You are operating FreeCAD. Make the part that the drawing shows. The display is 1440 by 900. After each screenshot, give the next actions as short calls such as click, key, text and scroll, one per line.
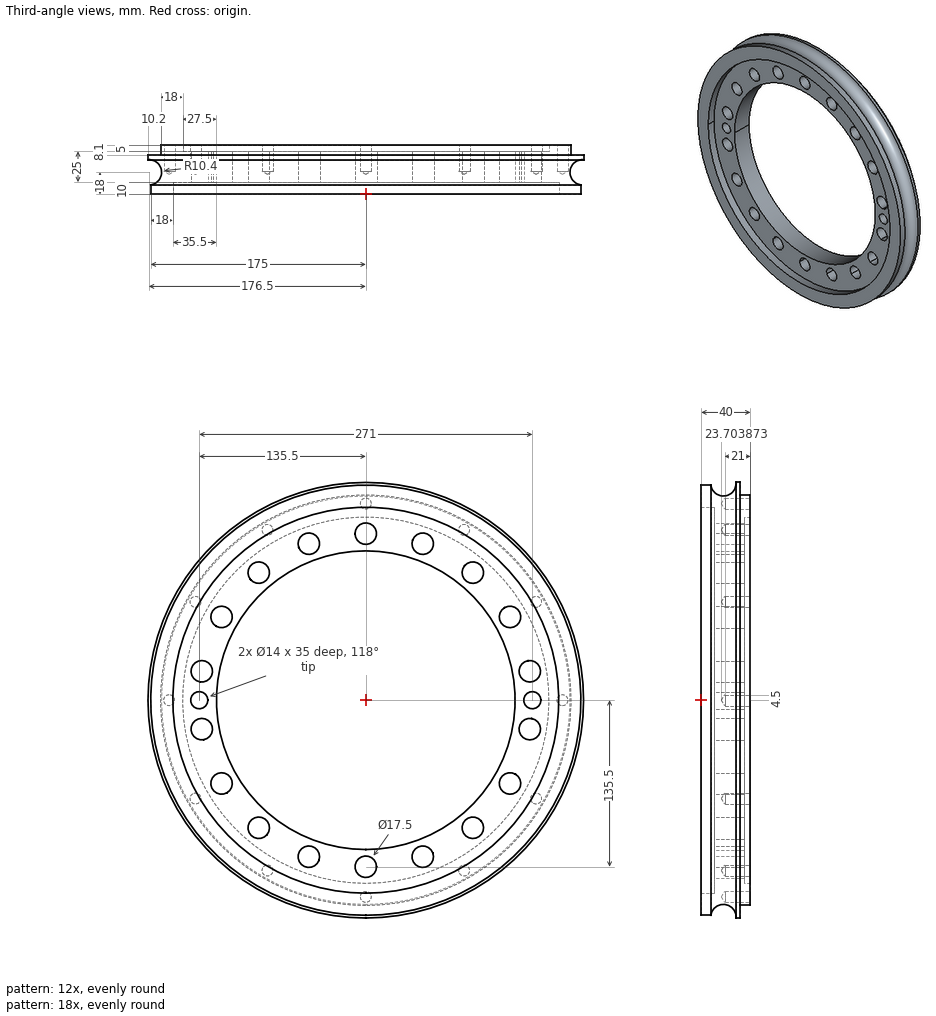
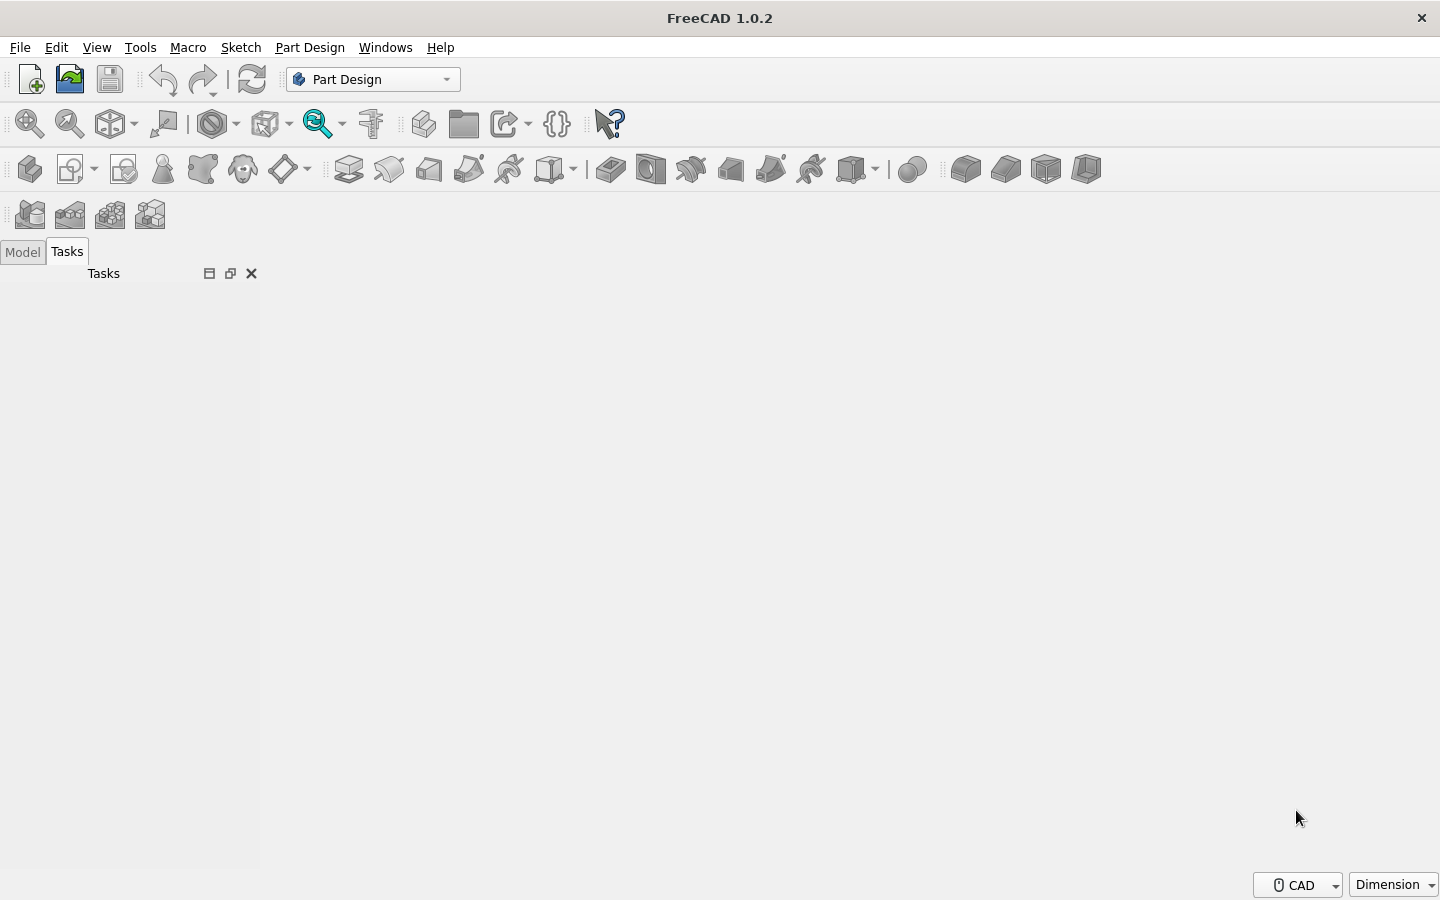
click(30, 80)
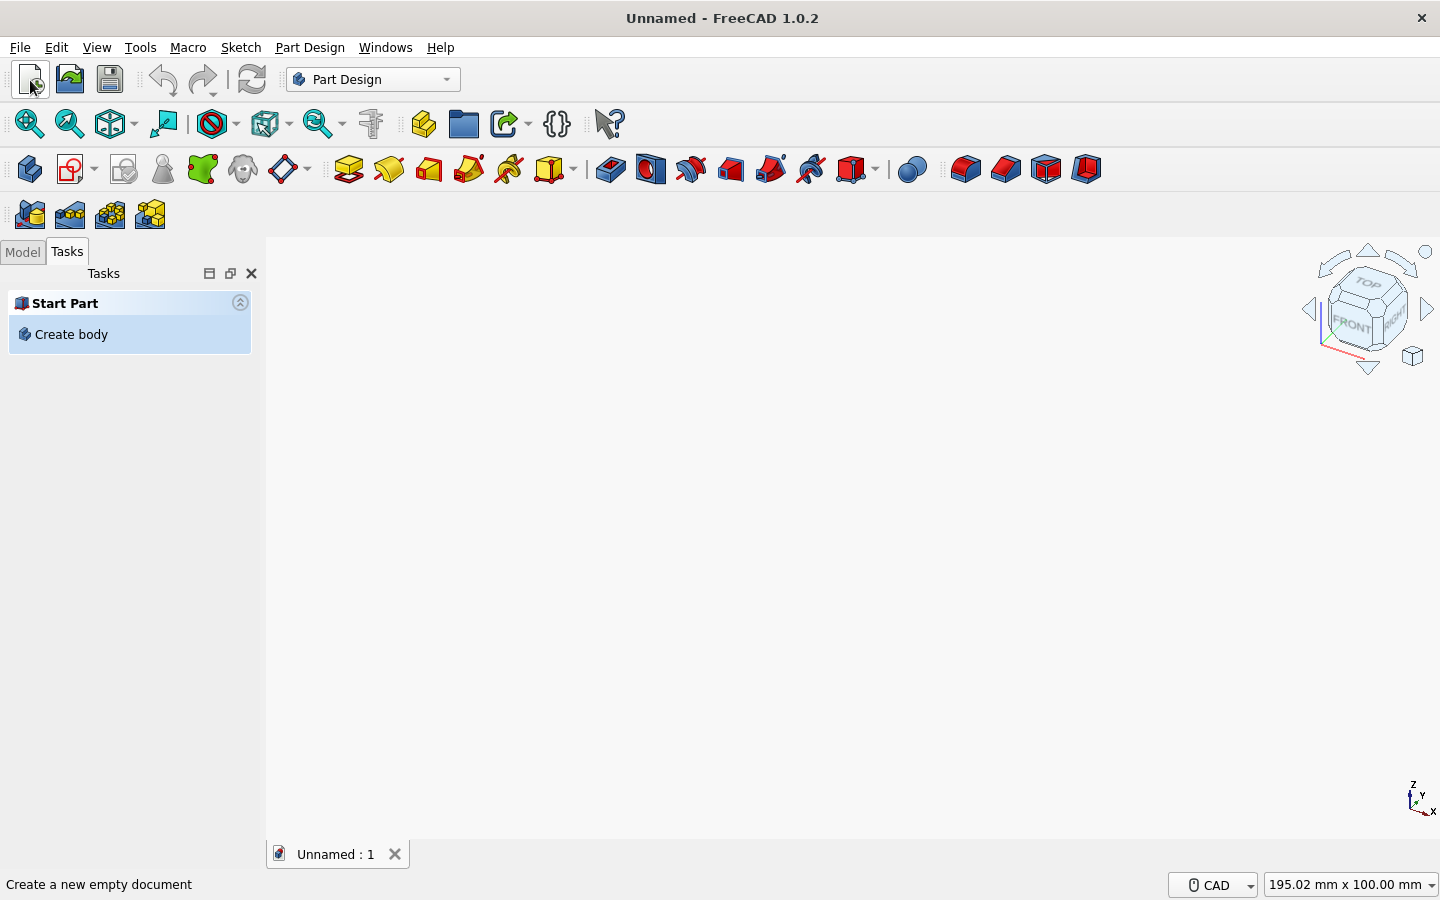
click(70, 170)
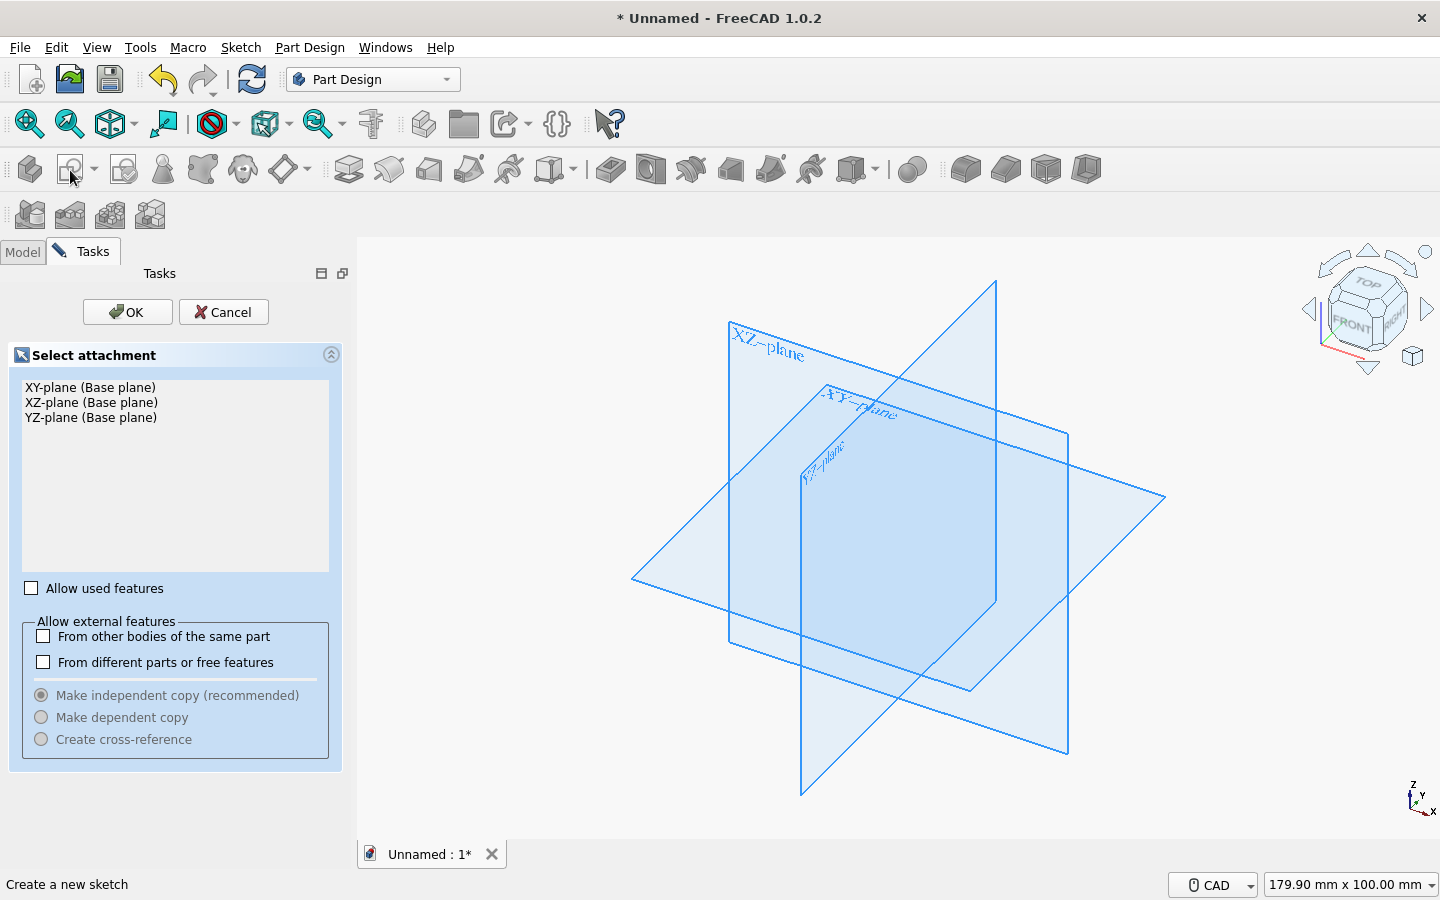
click(82, 388)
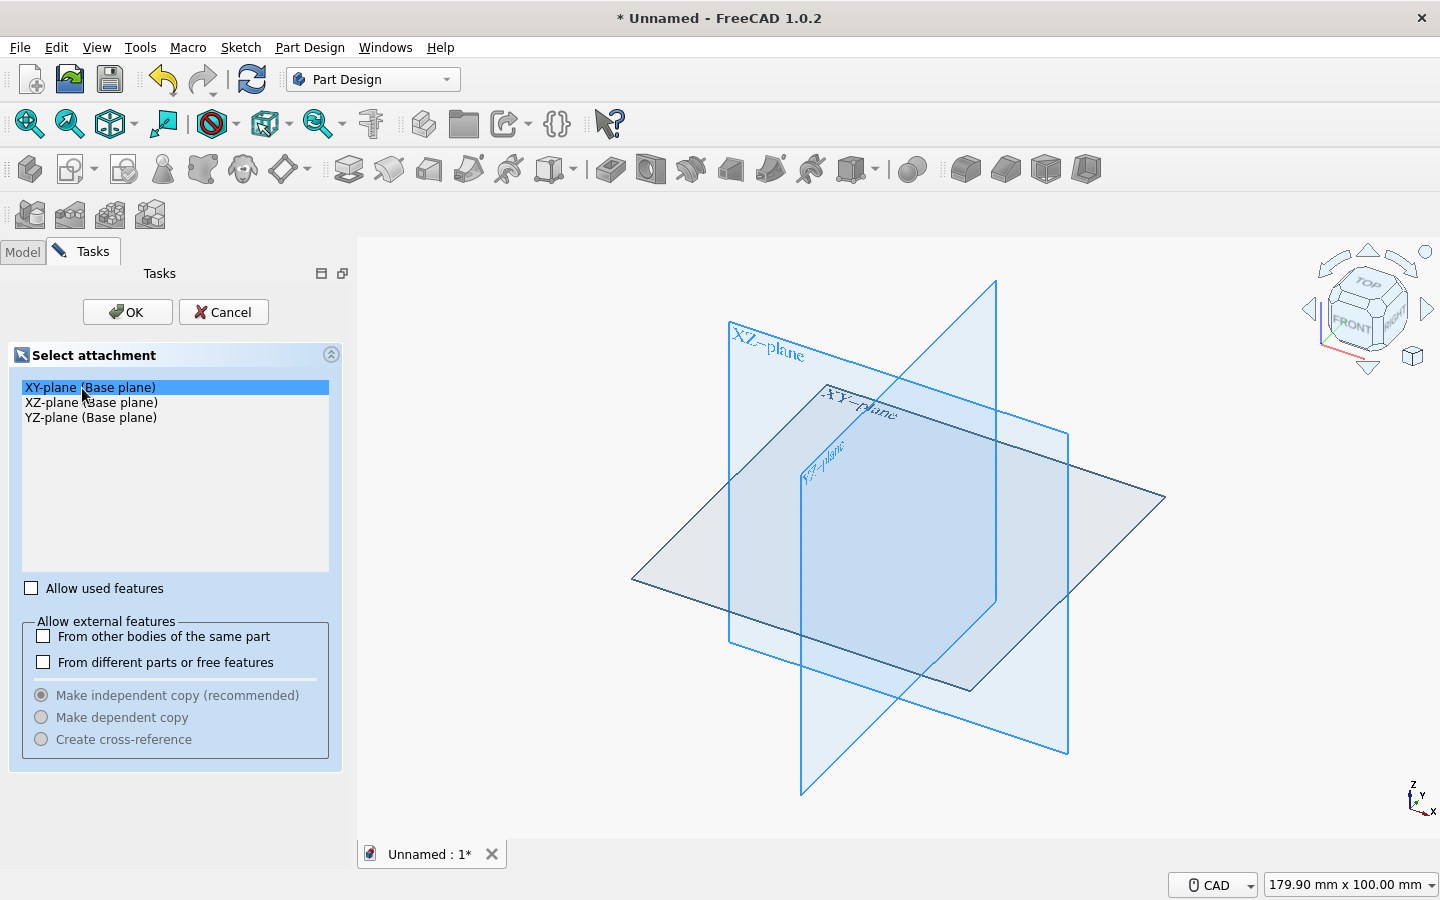
click(128, 312)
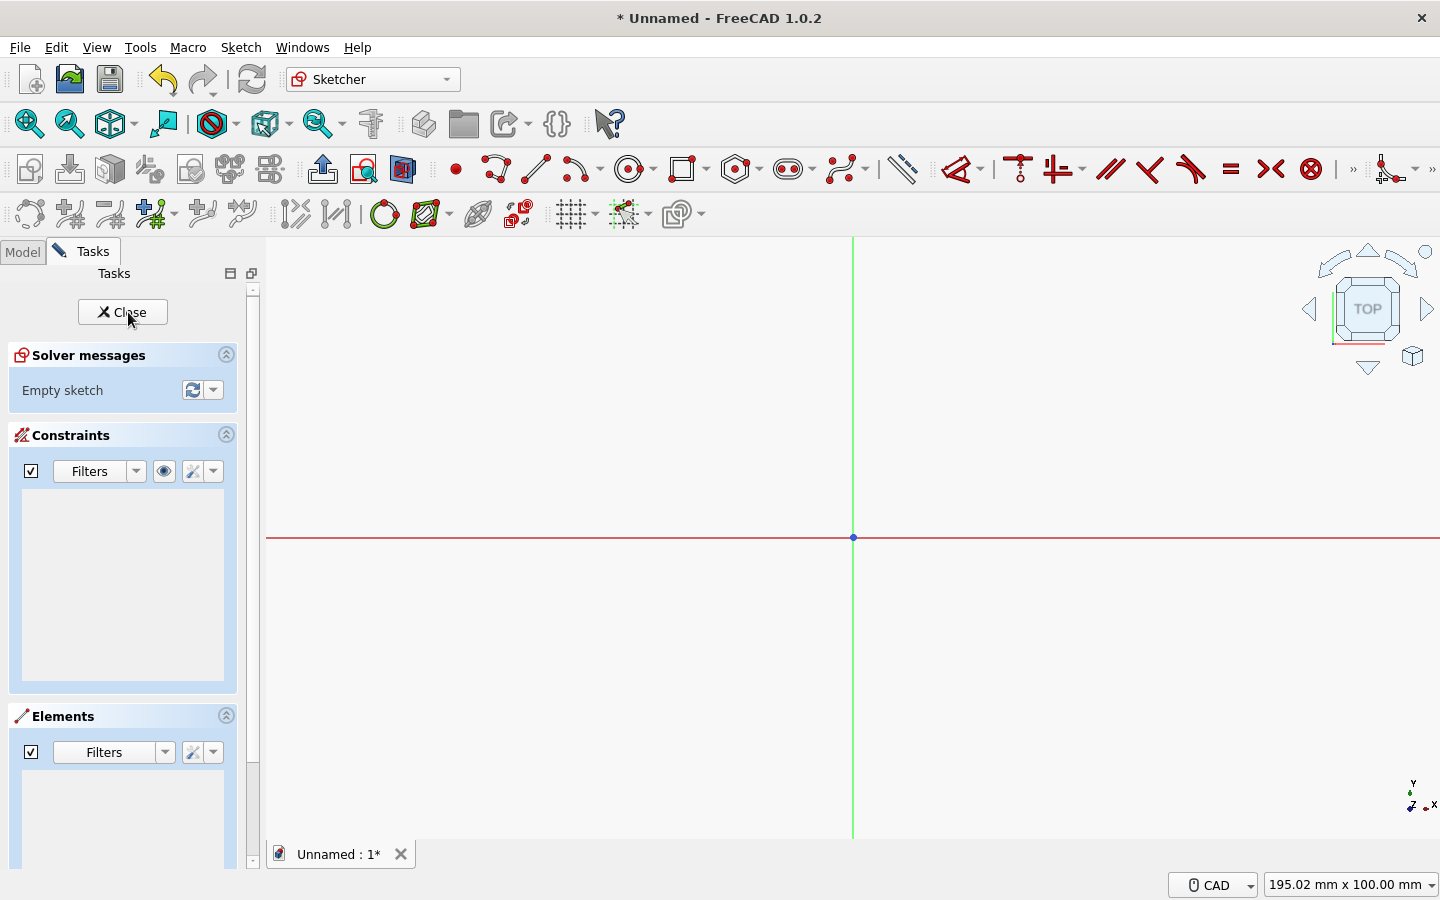
scroll(784, 538, down, 5)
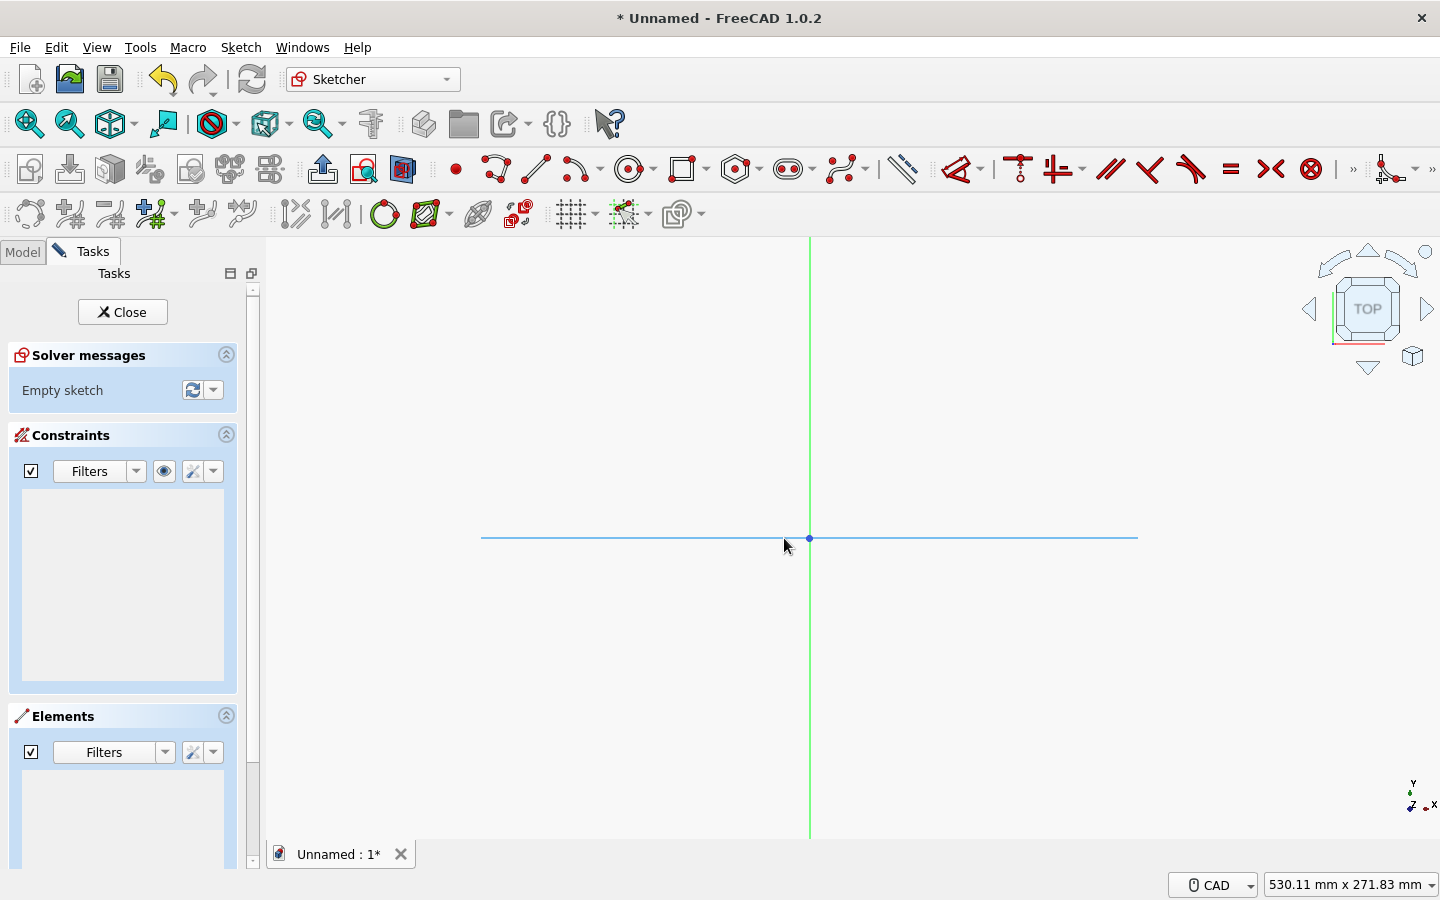
scroll(379, 480, up, 7)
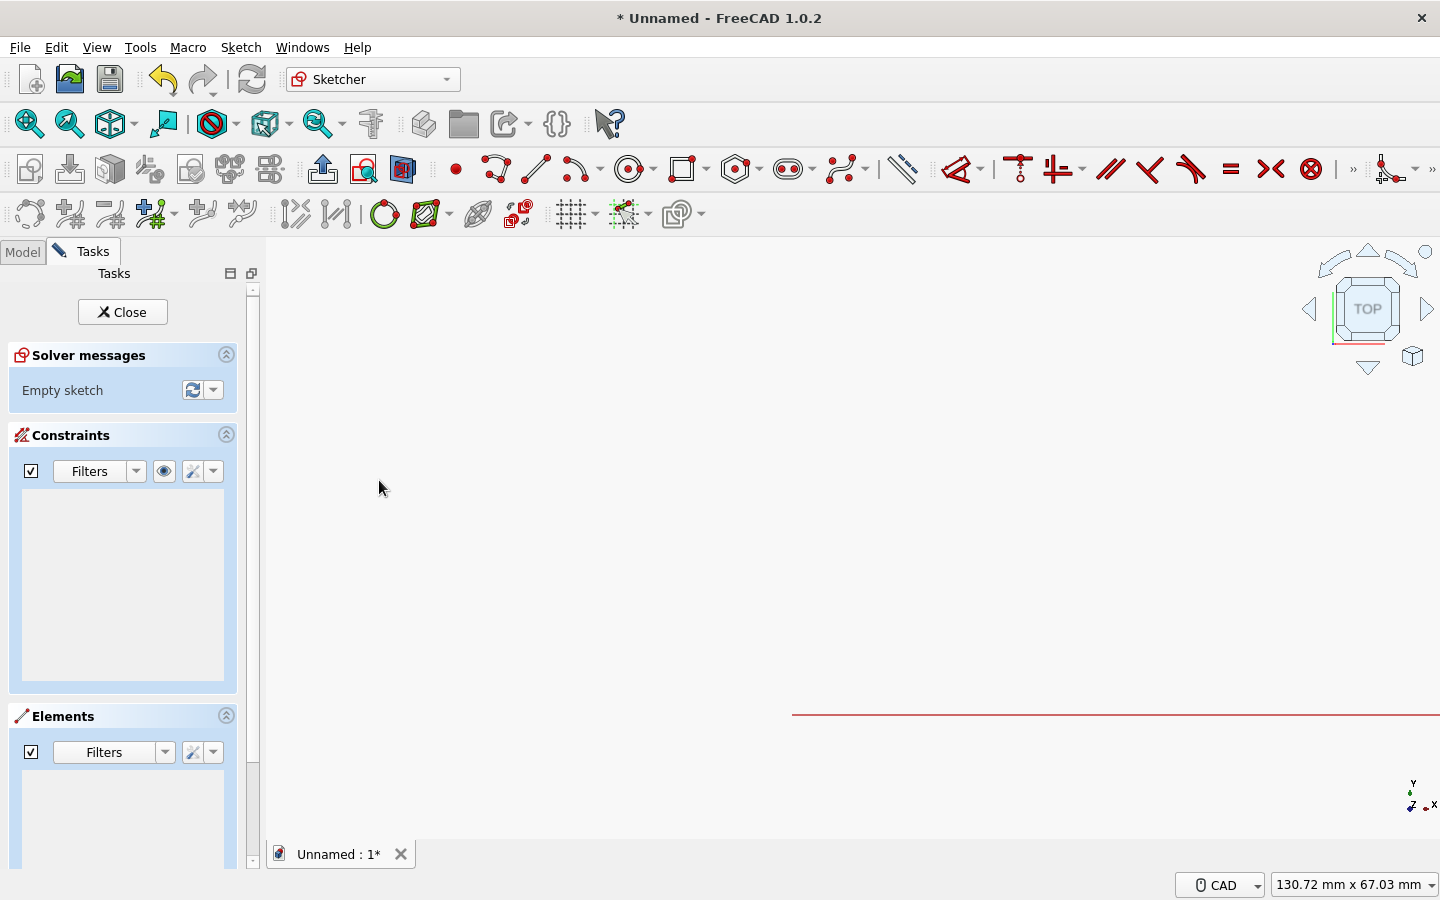
click(496, 170)